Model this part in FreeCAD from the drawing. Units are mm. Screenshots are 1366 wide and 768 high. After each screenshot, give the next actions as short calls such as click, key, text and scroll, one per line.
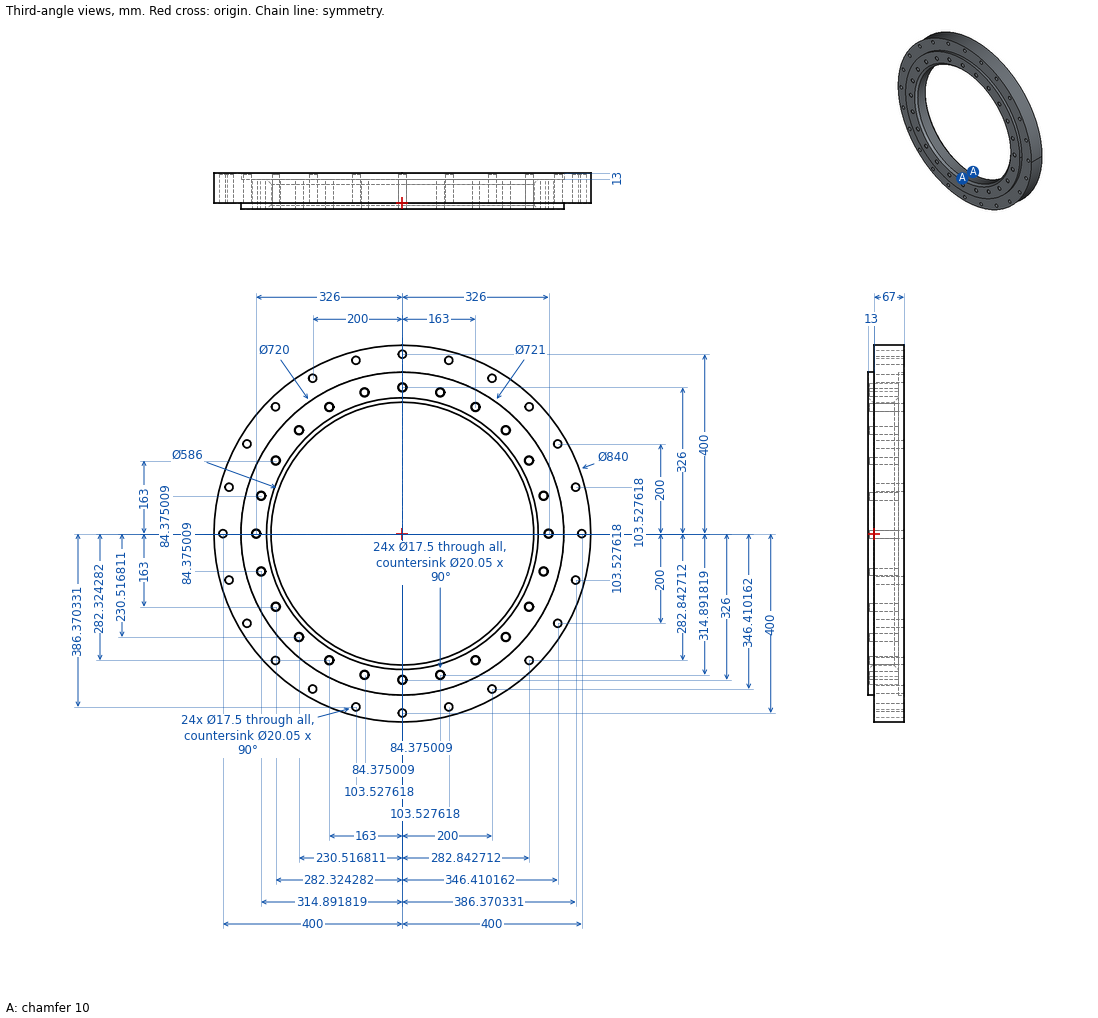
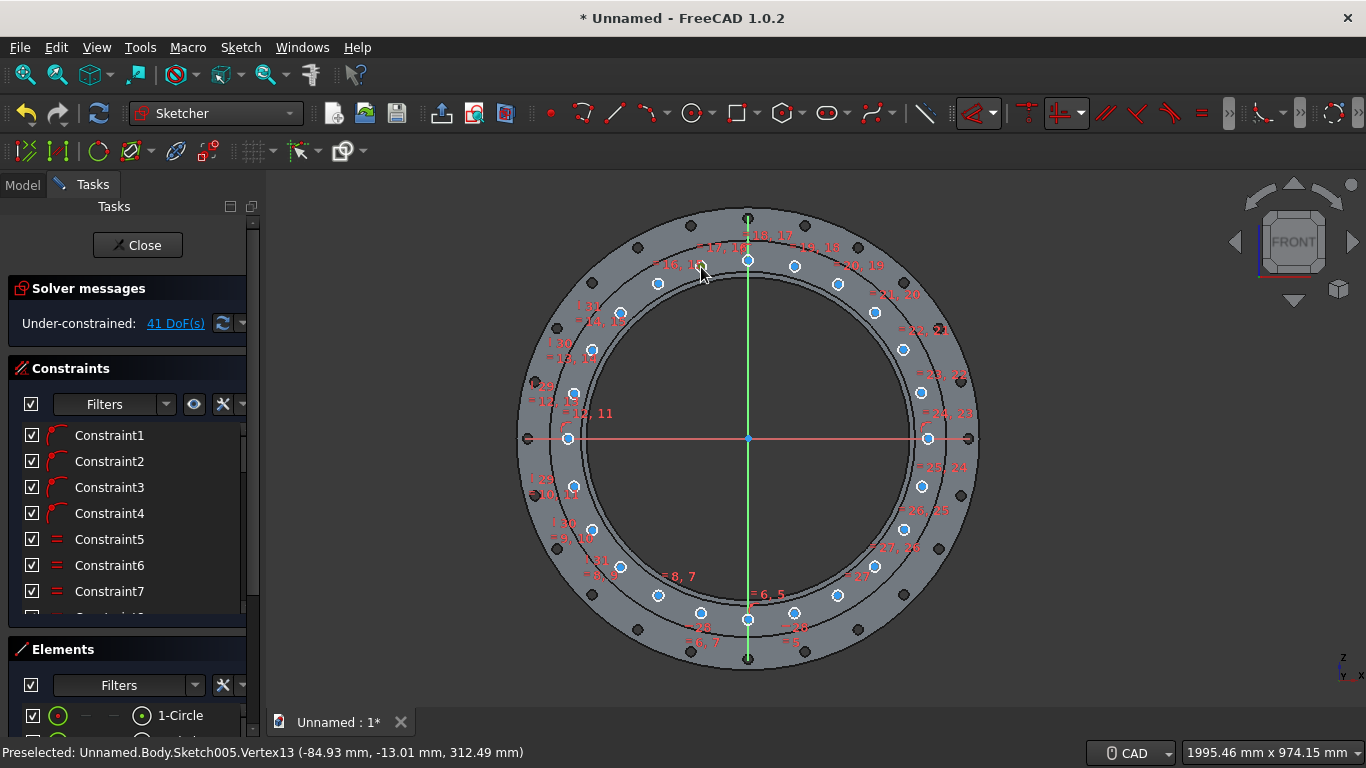
click(795, 266)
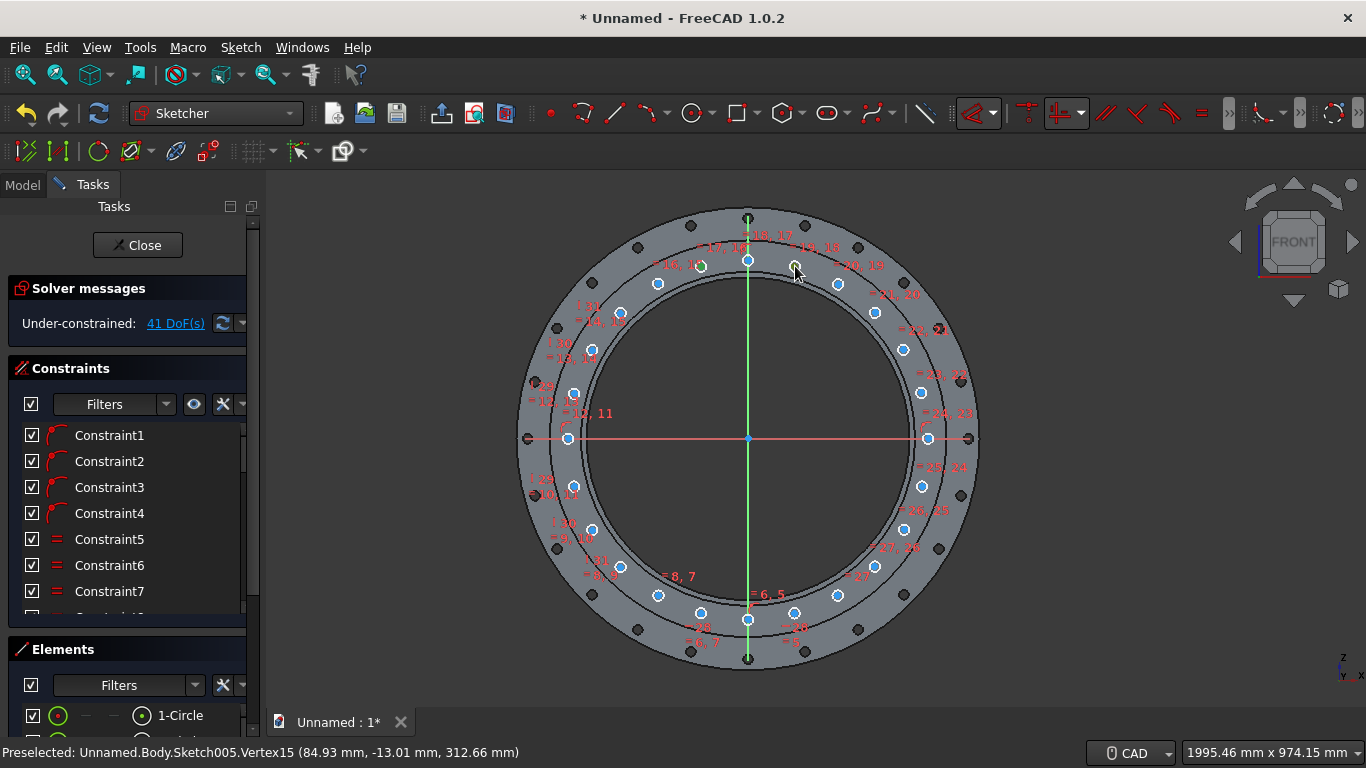
key(h)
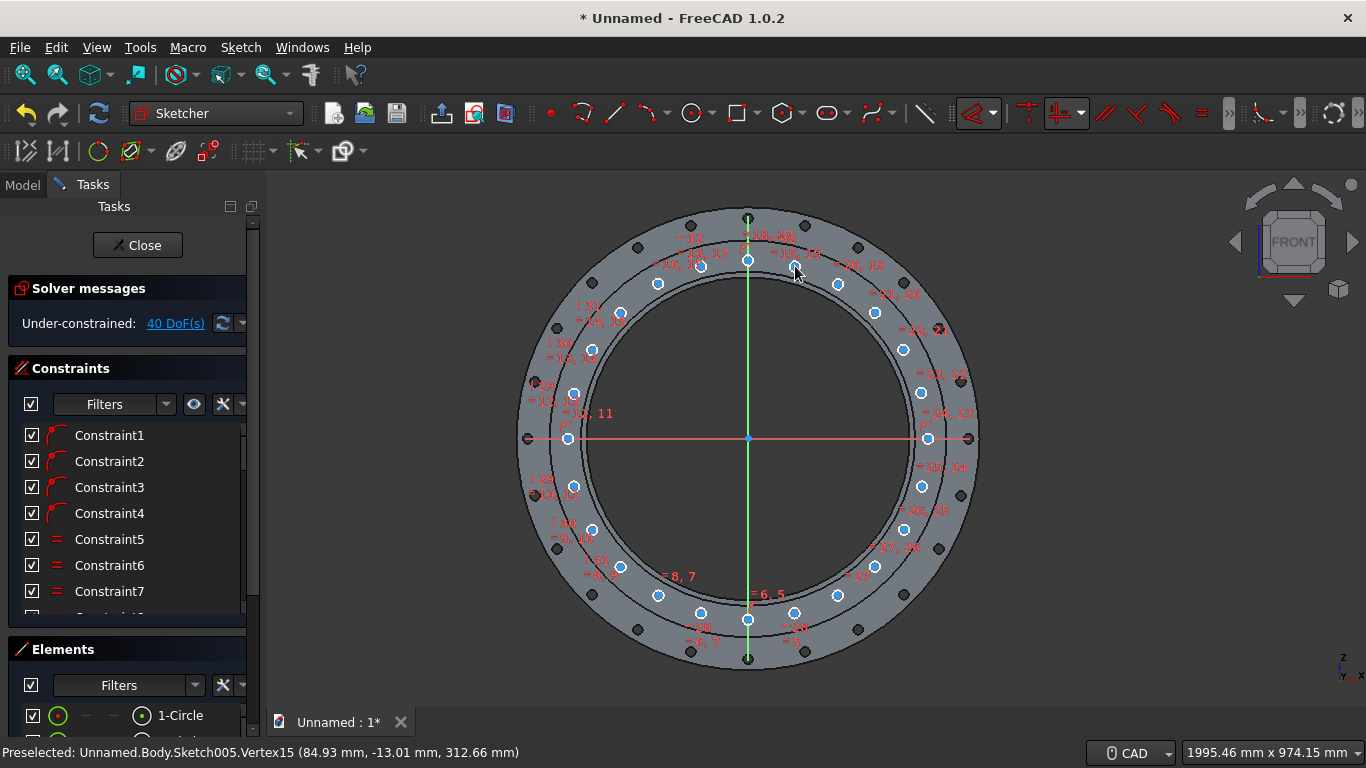
click(658, 284)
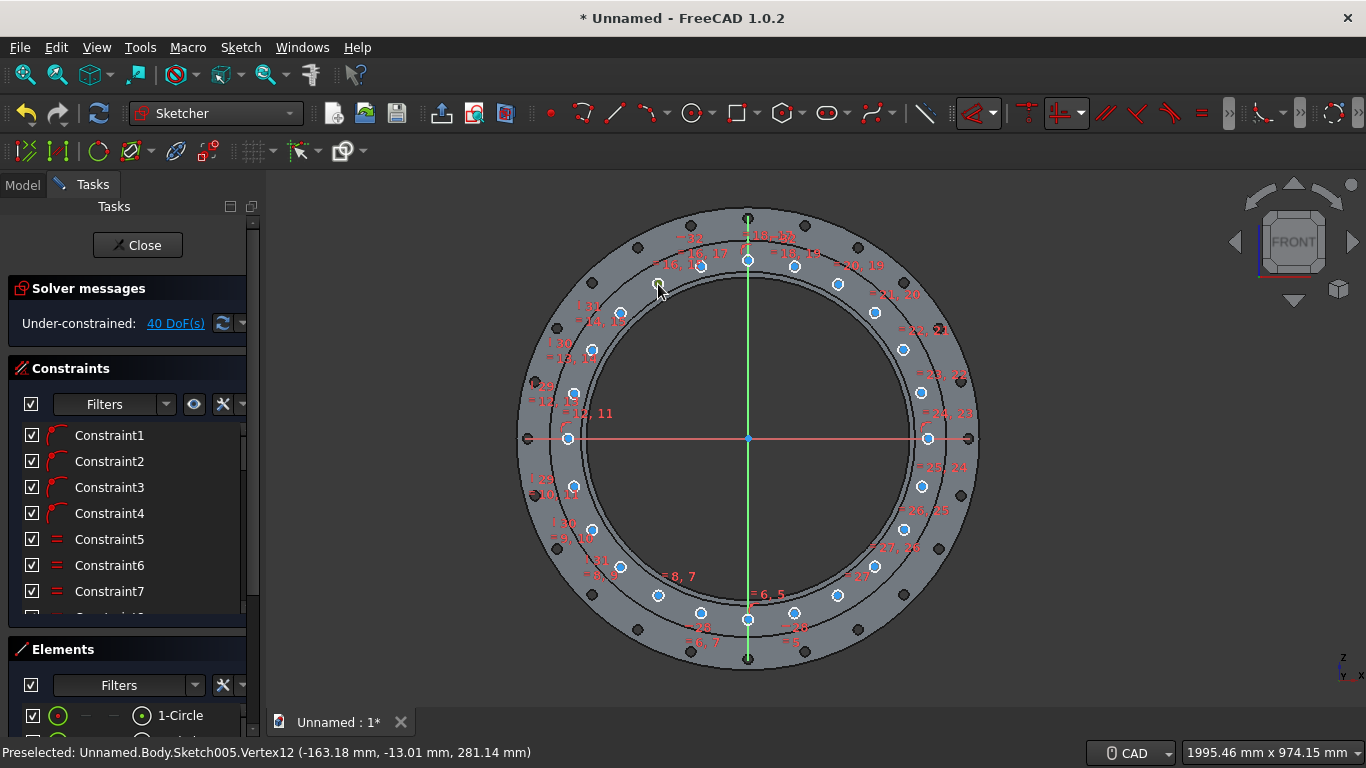
click(838, 284)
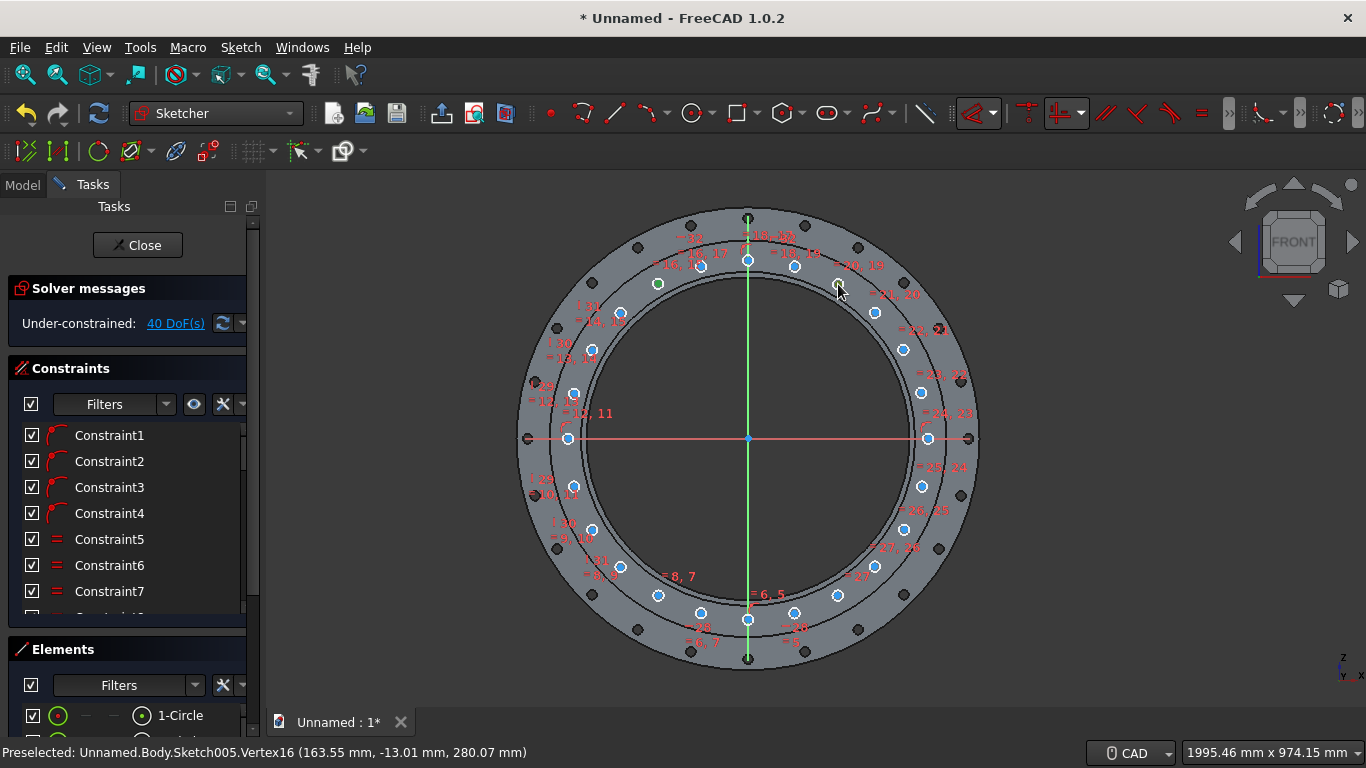
key(h)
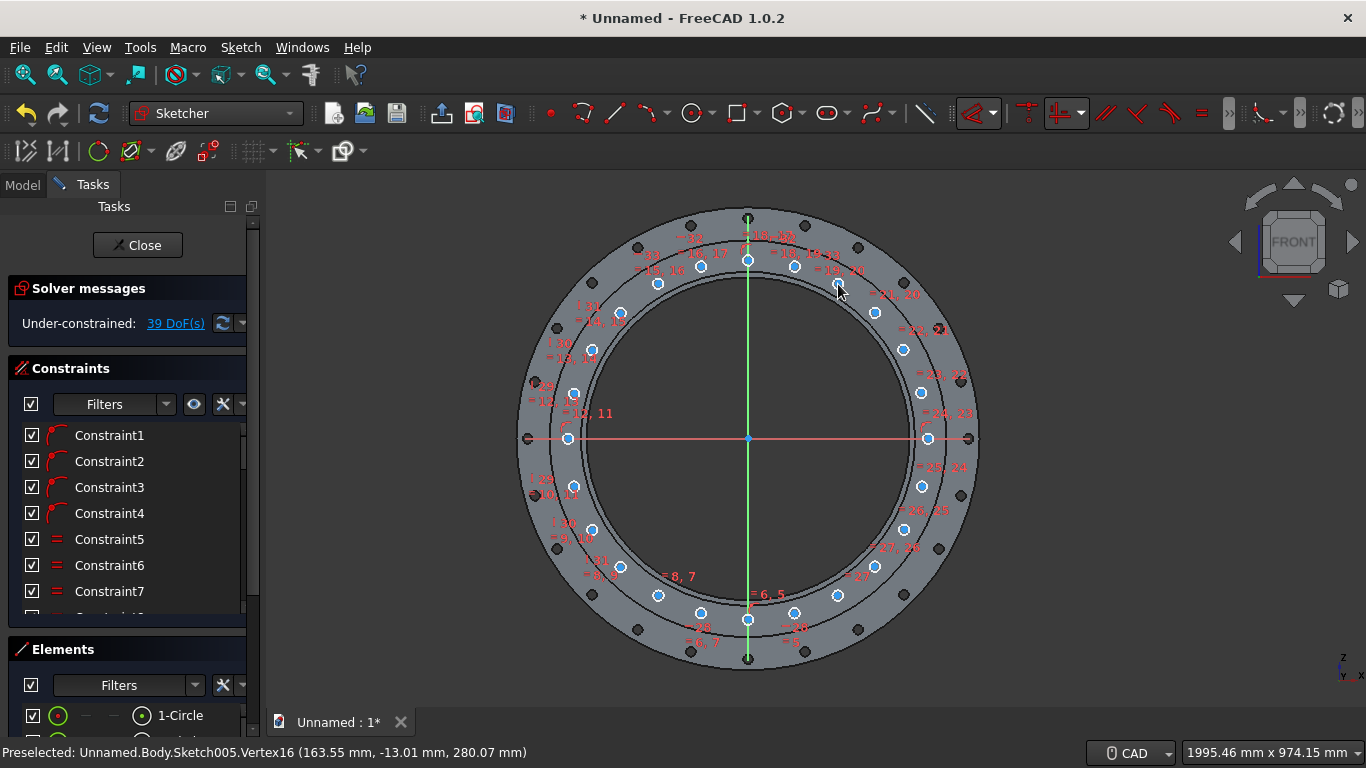
scroll(621, 313, up, 4)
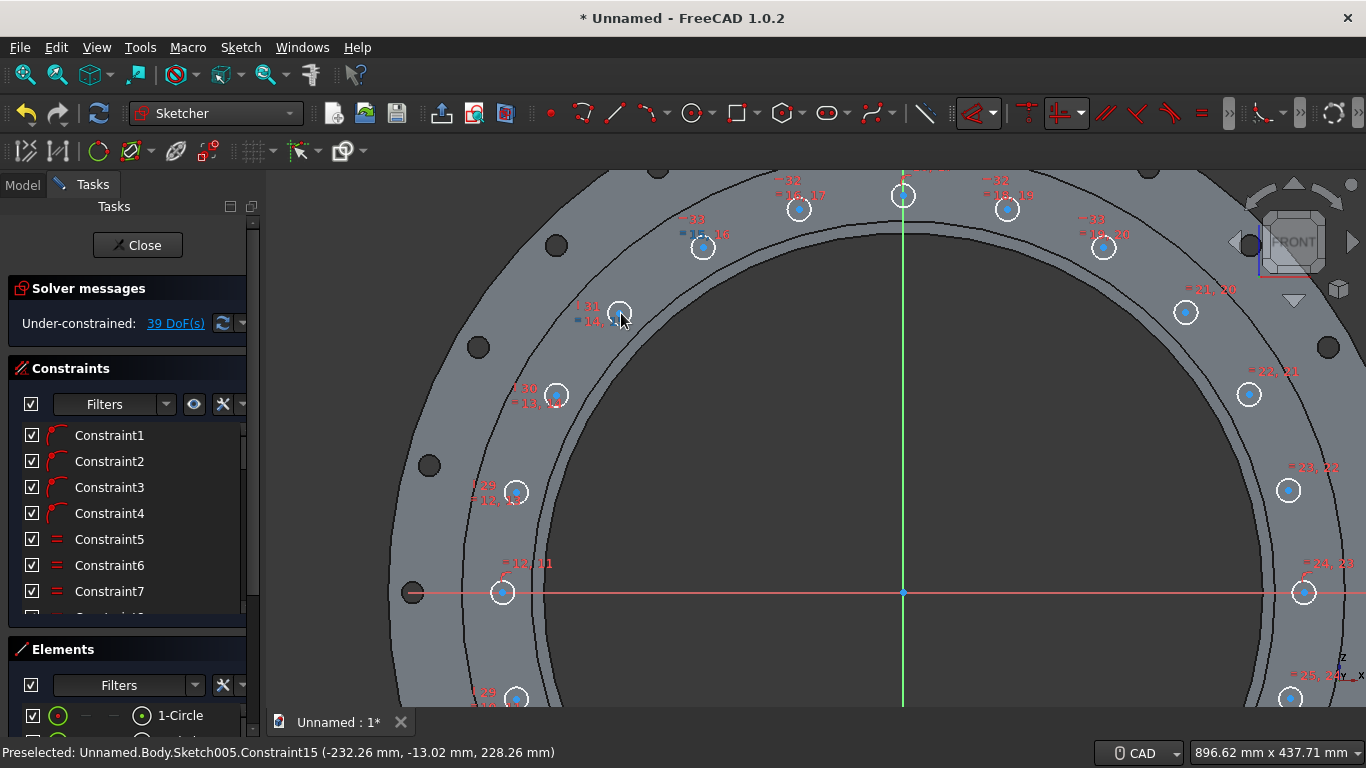
scroll(620, 313, up, 4)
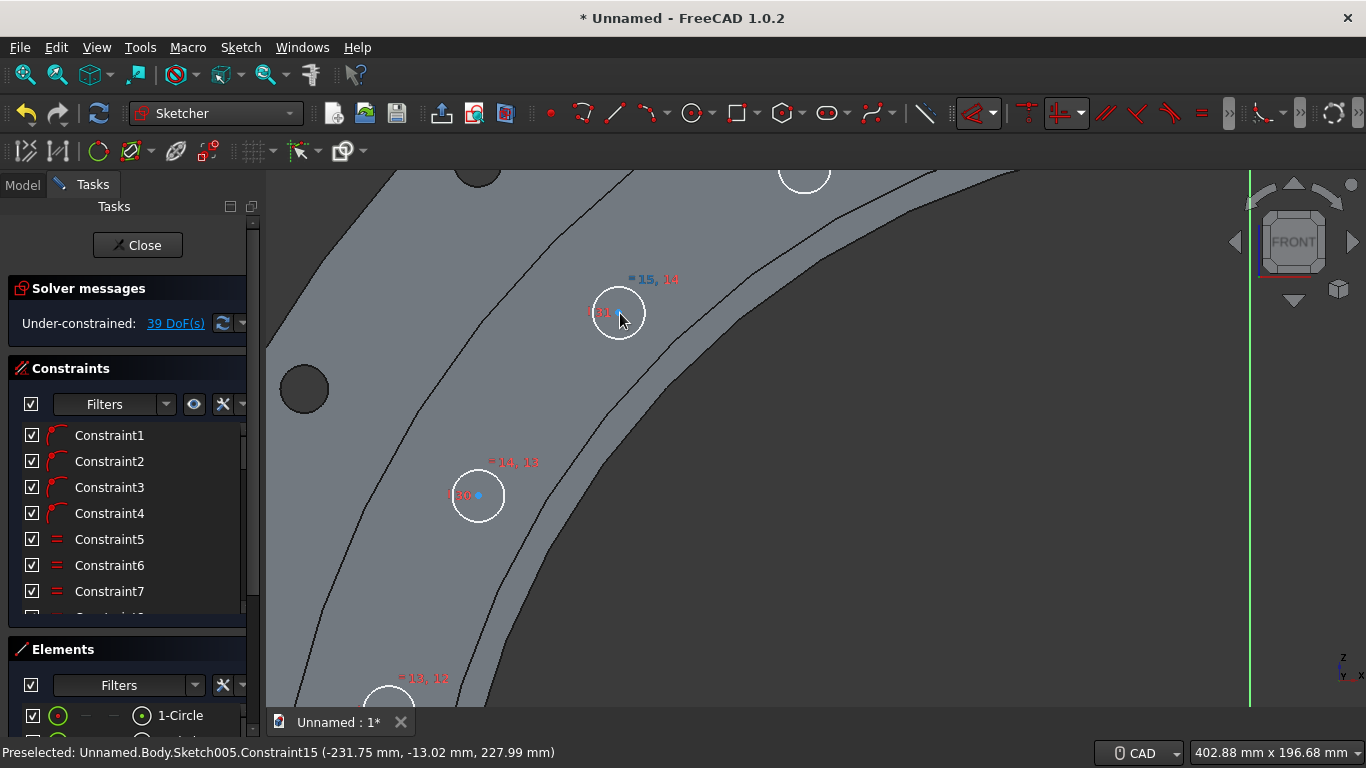
click(619, 313)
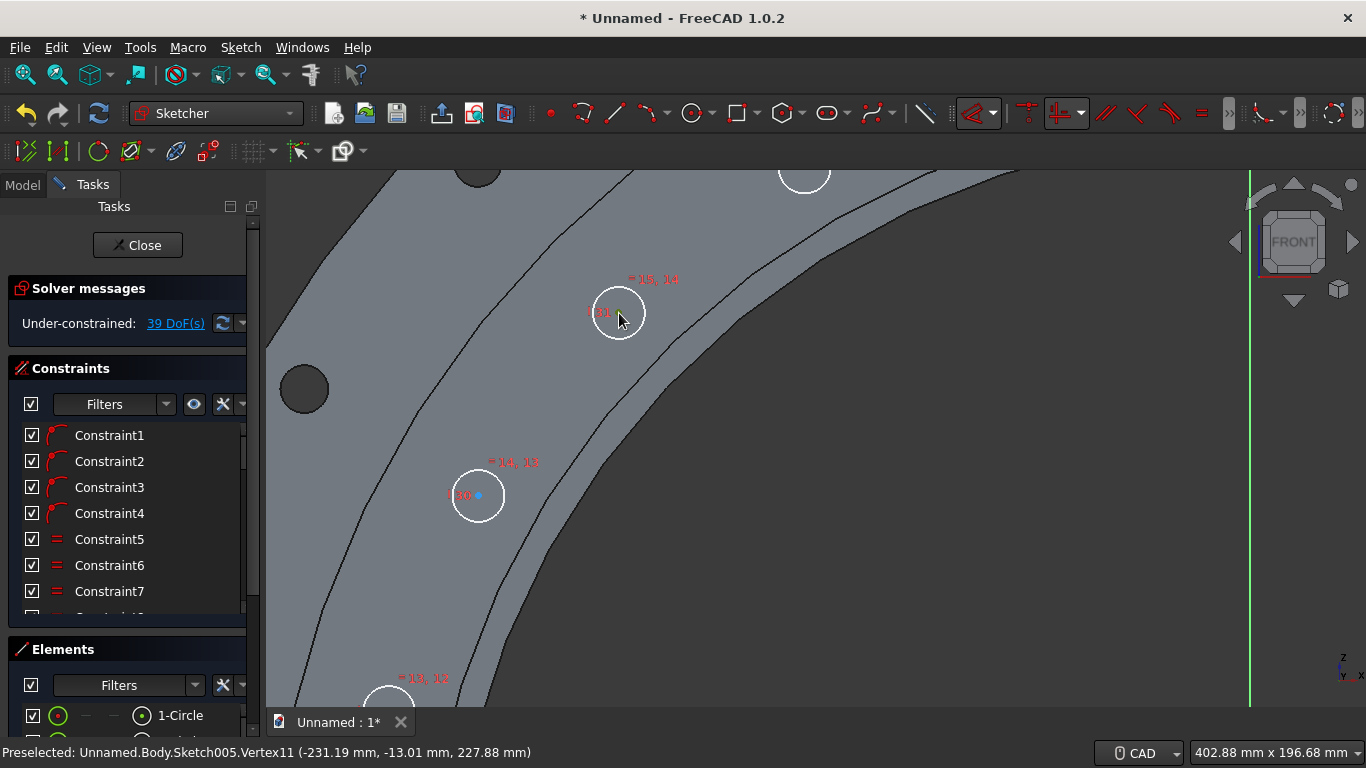
scroll(620, 313, down, 8)